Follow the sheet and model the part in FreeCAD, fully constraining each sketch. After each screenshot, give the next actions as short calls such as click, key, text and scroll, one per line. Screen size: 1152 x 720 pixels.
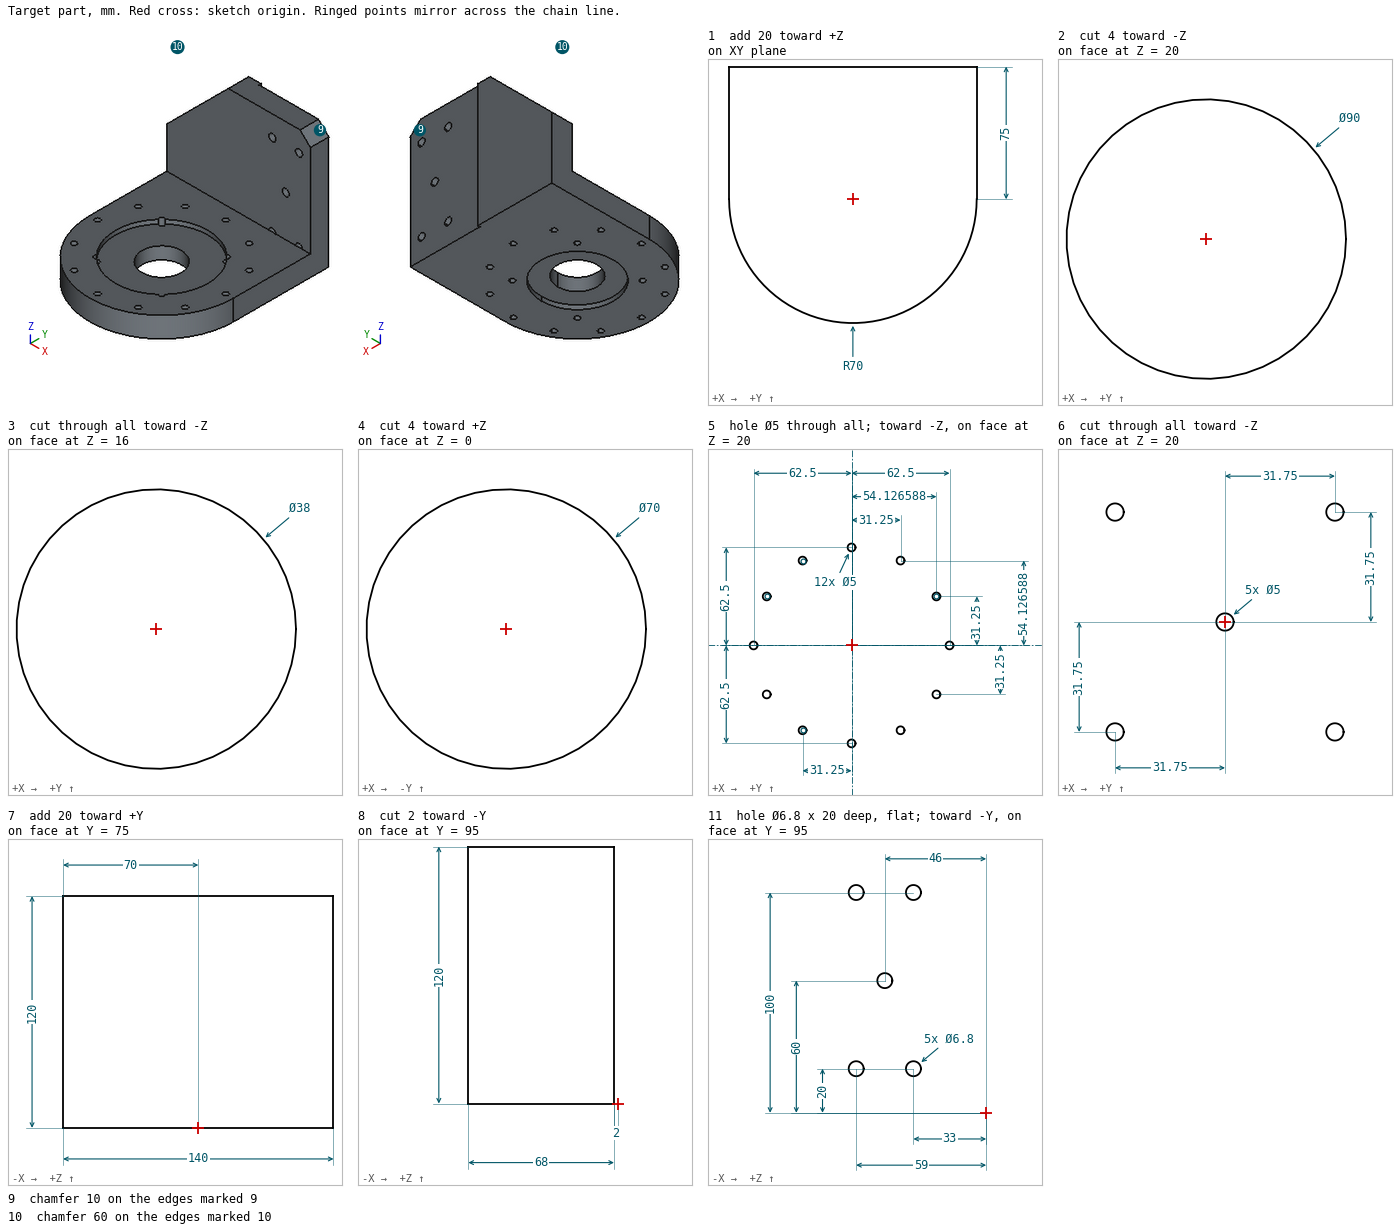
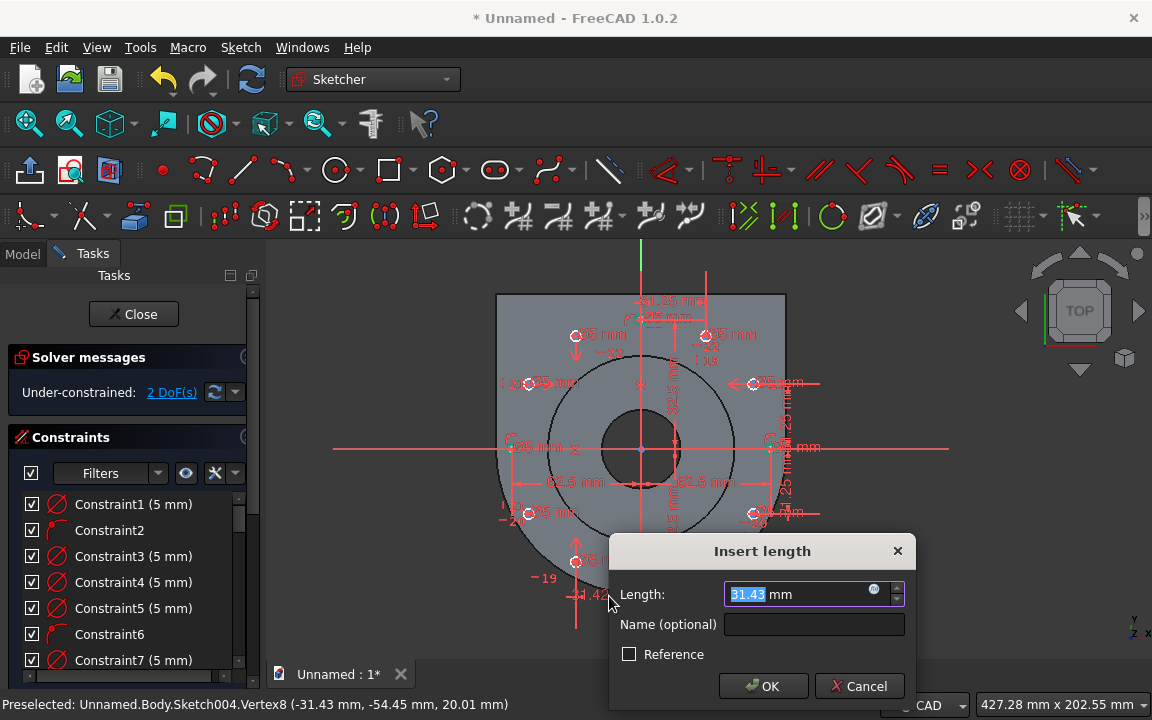
text(31.25)
key(Return)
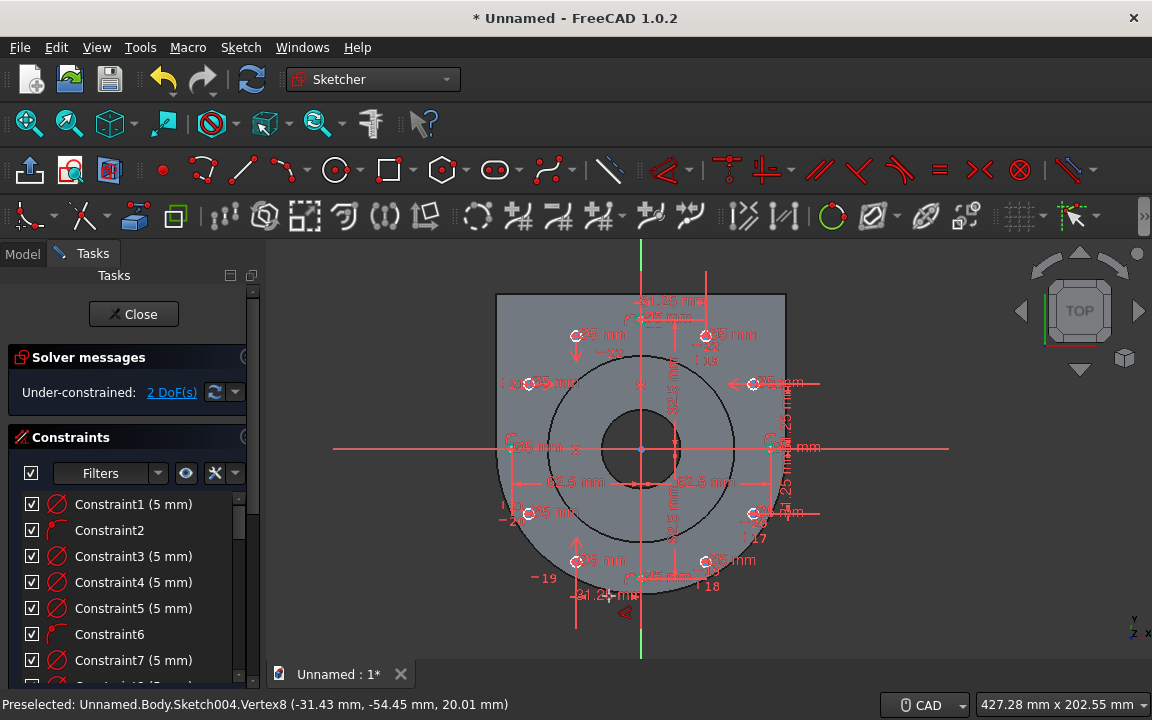
click(706, 336)
click(740, 353)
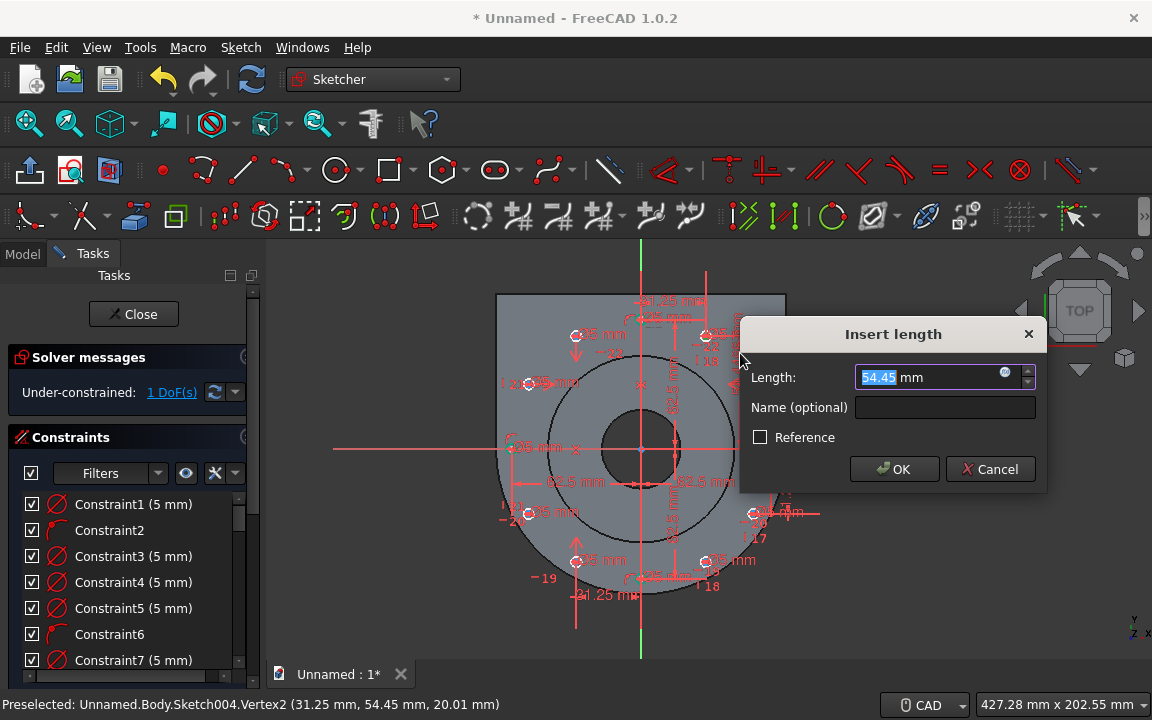
text(54.126588)
key(Return)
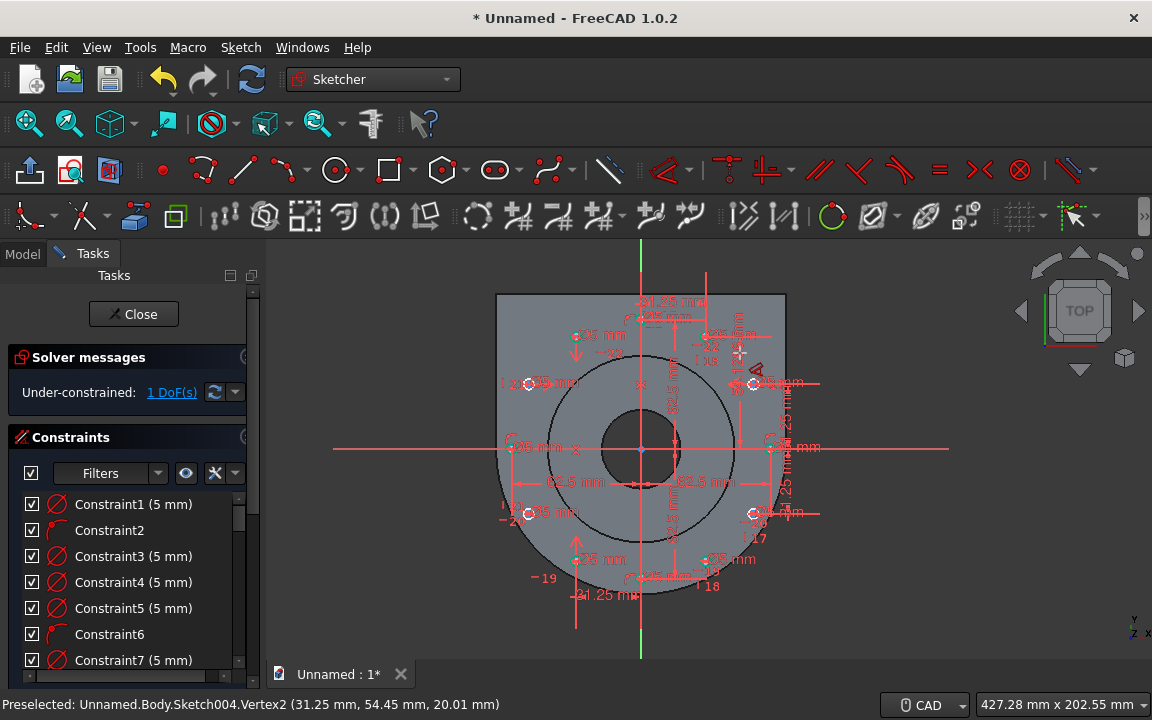
click(754, 384)
click(658, 350)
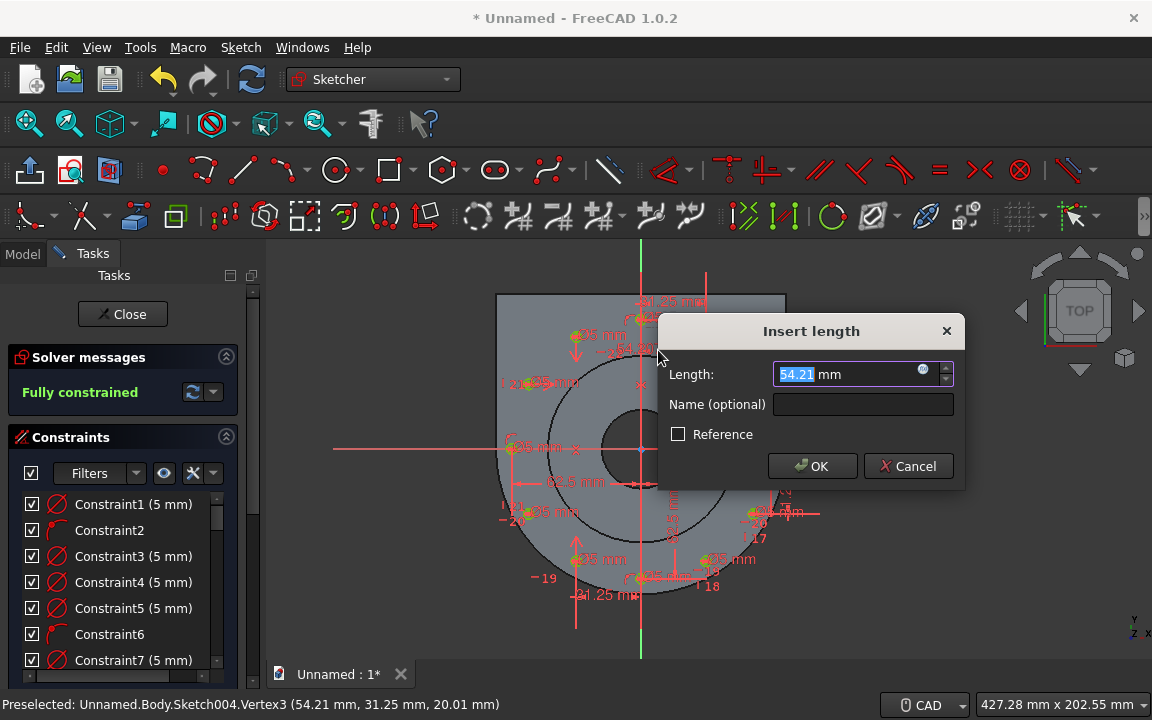
text(54.126588)
key(Return)
key(Escape)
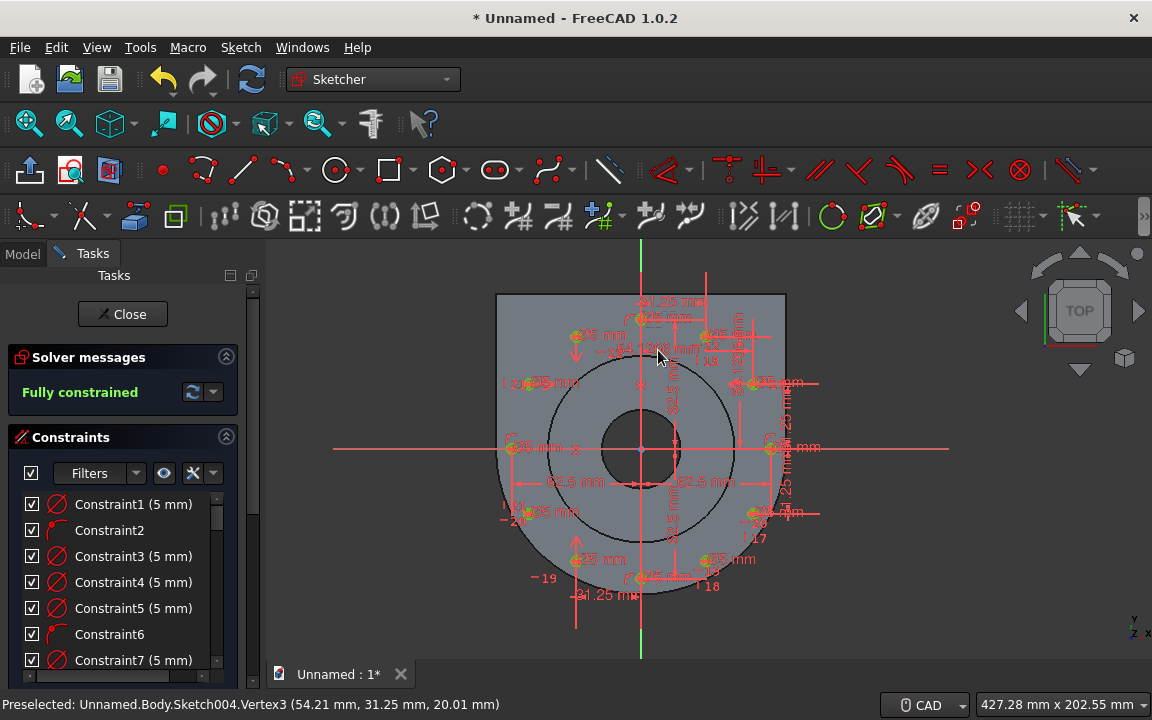
click(123, 314)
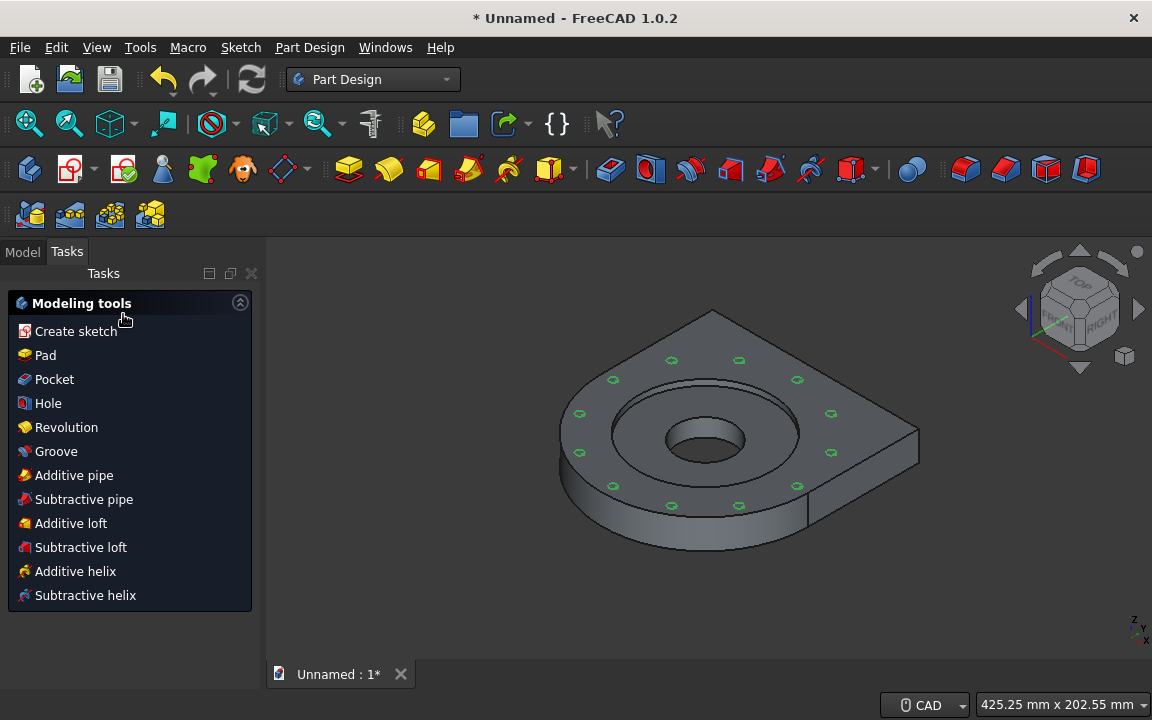
click(652, 170)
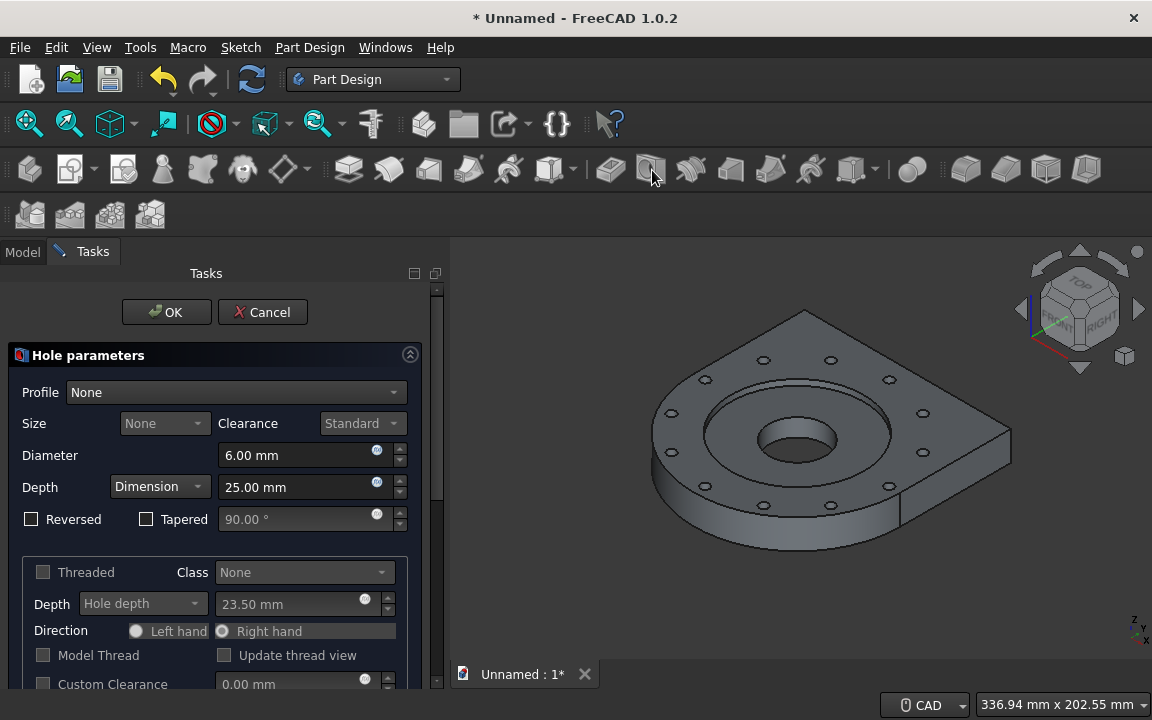
triple_click(305, 455)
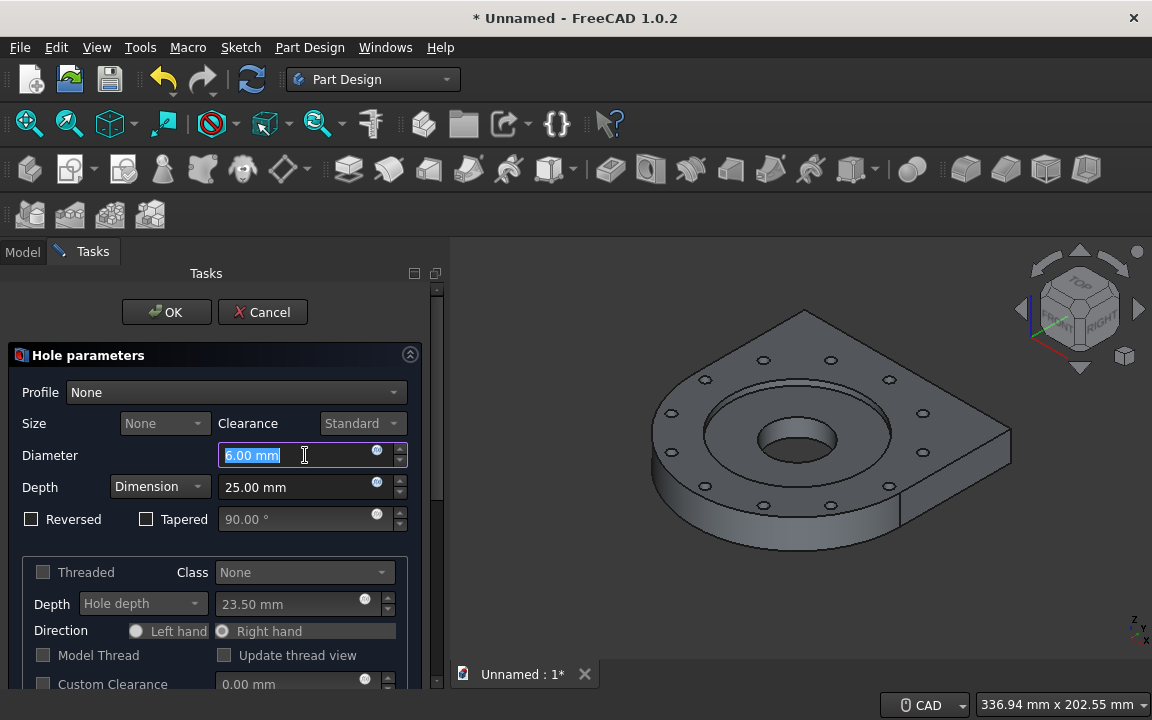
text(5)
key(Tab)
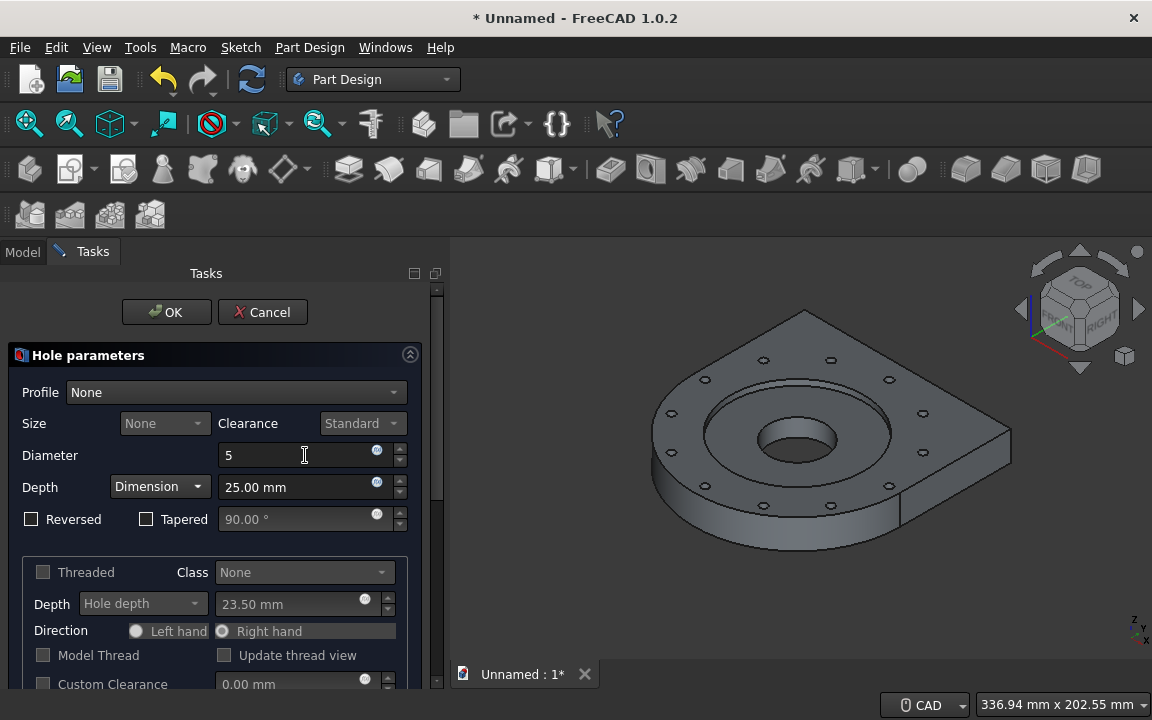
click(161, 486)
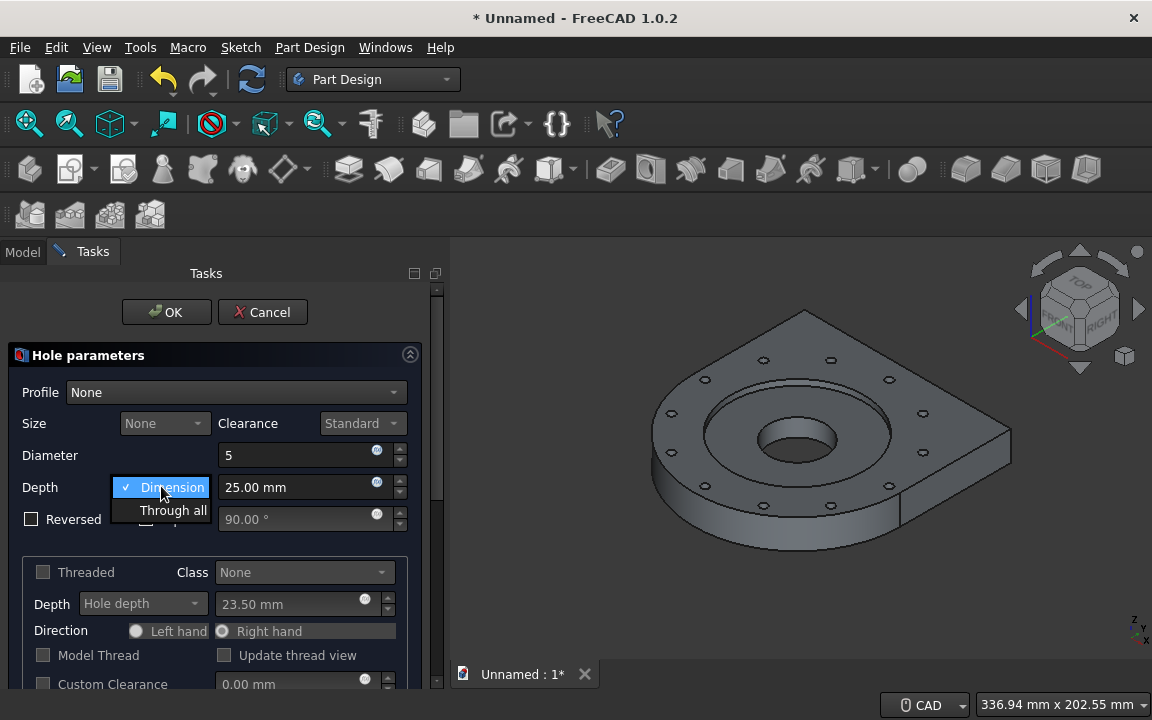
click(160, 510)